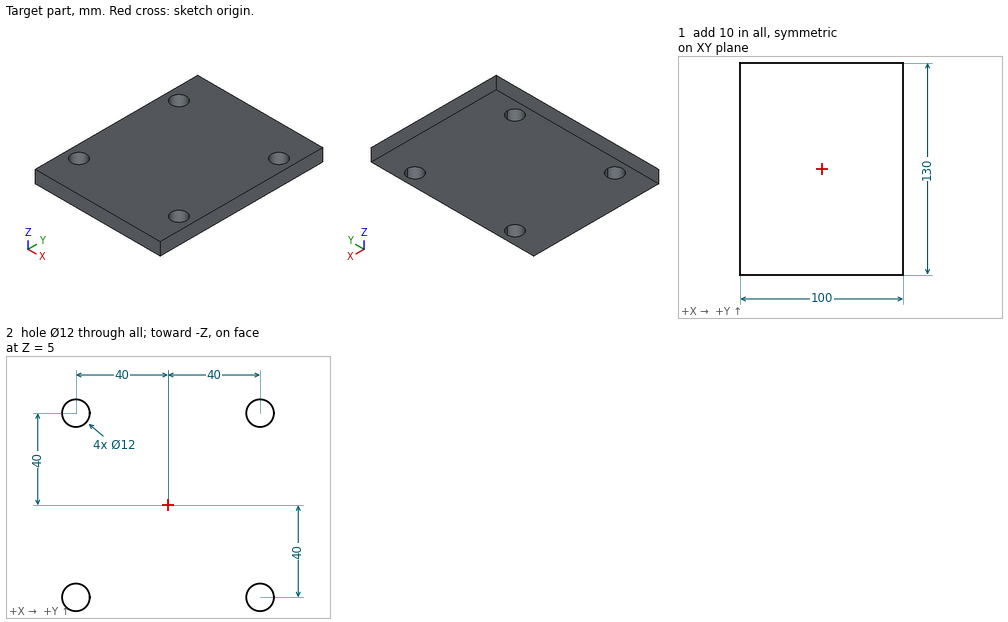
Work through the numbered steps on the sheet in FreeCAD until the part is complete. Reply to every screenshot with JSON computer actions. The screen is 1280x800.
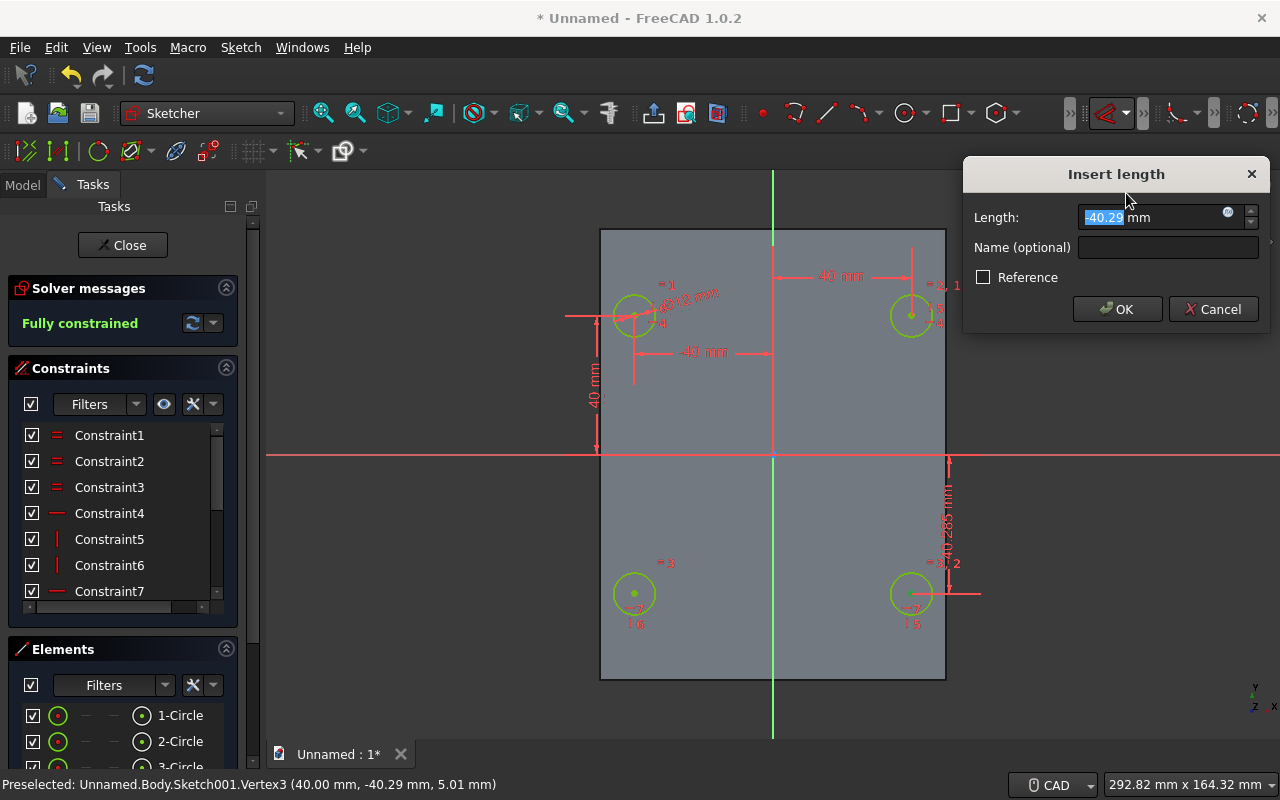
{"action": "type", "text": "-40"}
{"action": "key", "text": "Return"}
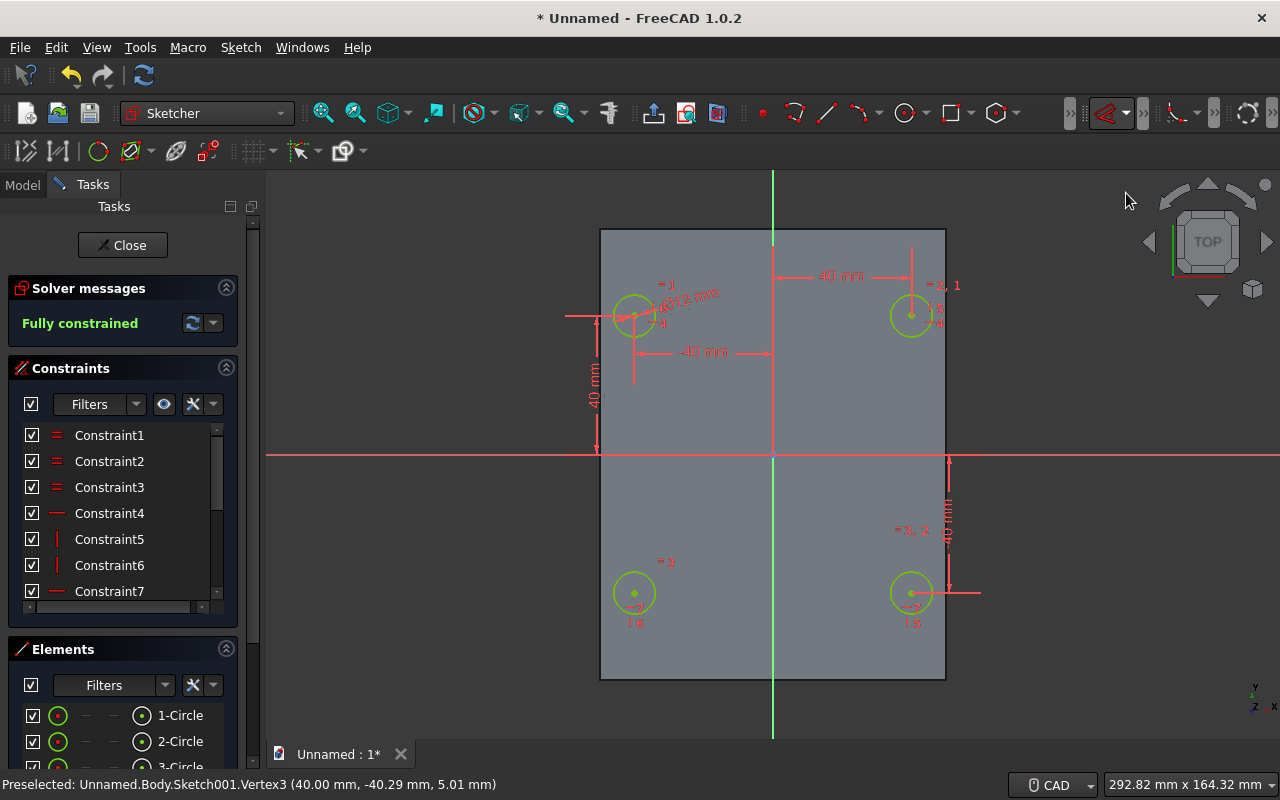
{"action": "left_click", "coordinate": [123, 245]}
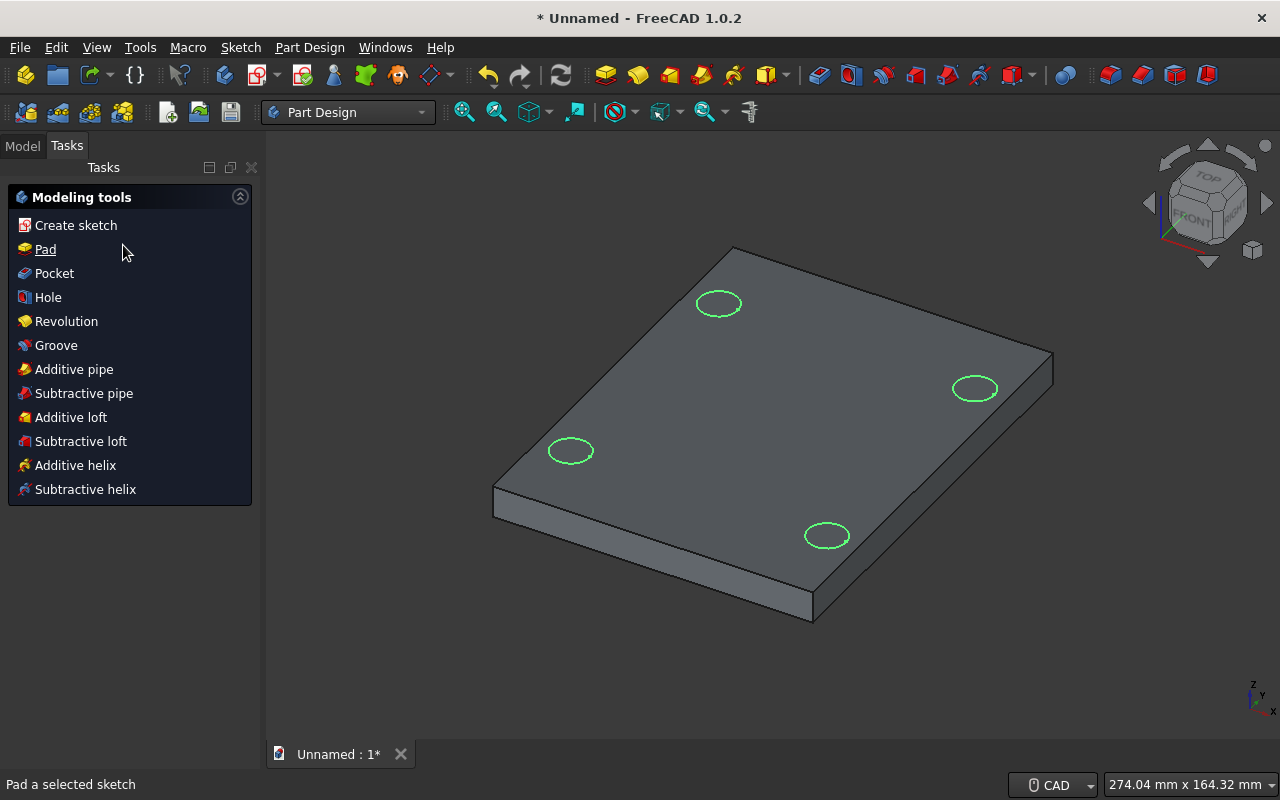
{"action": "left_click", "coordinate": [852, 76]}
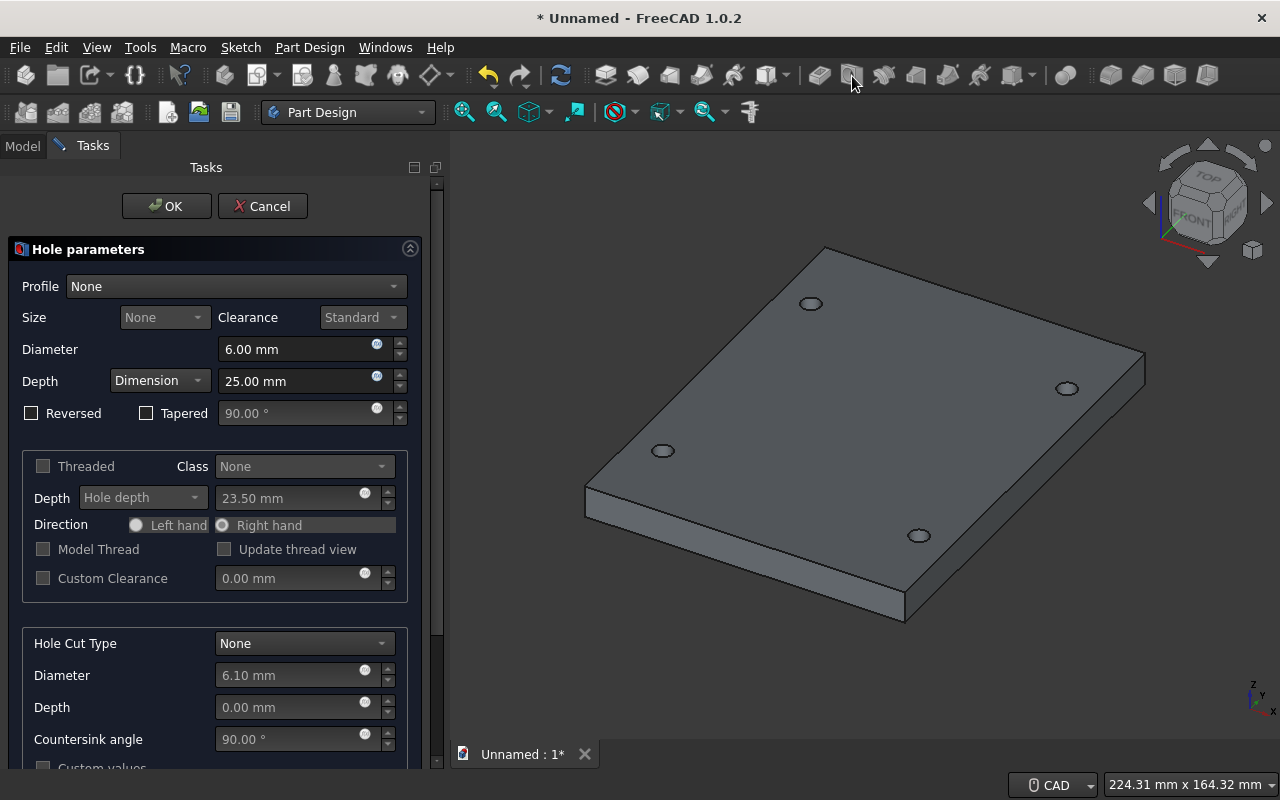
{"action": "triple_click", "coordinate": [305, 349]}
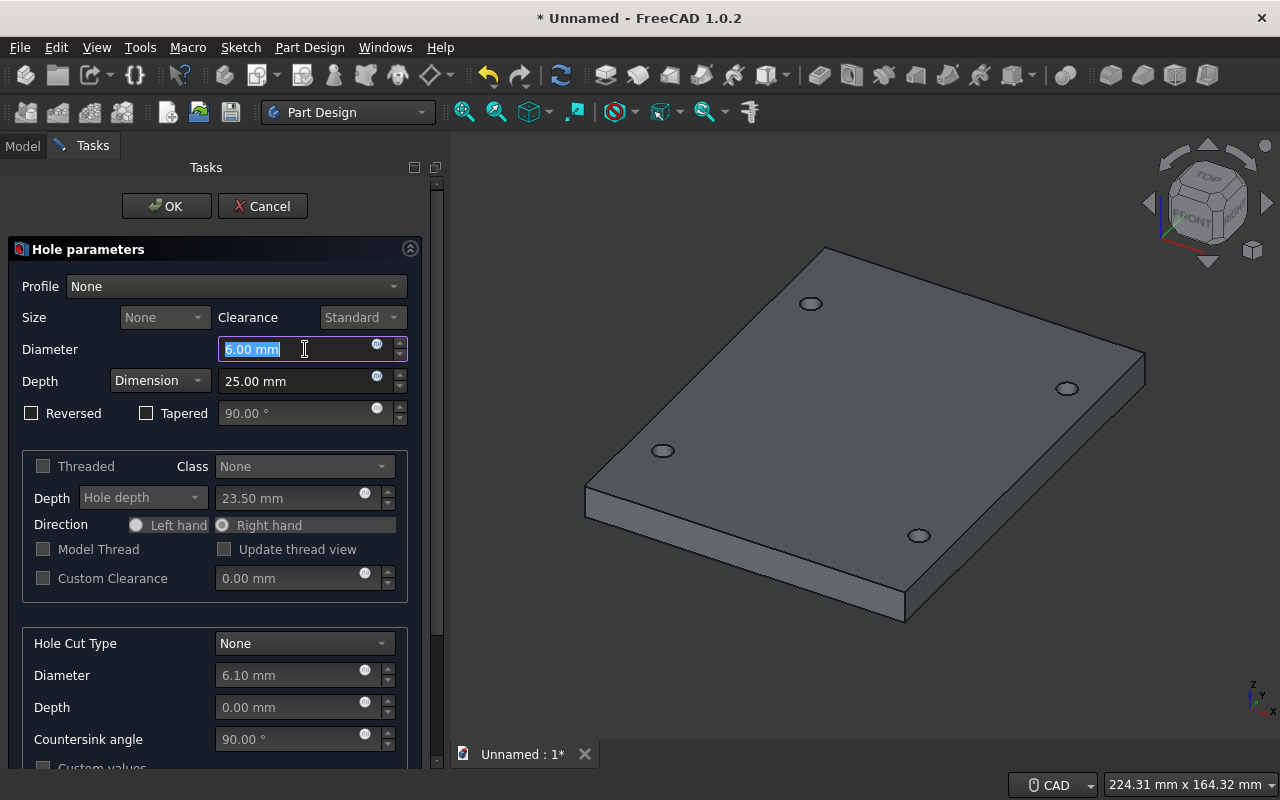
{"action": "type", "text": "12"}
{"action": "key", "text": "Tab"}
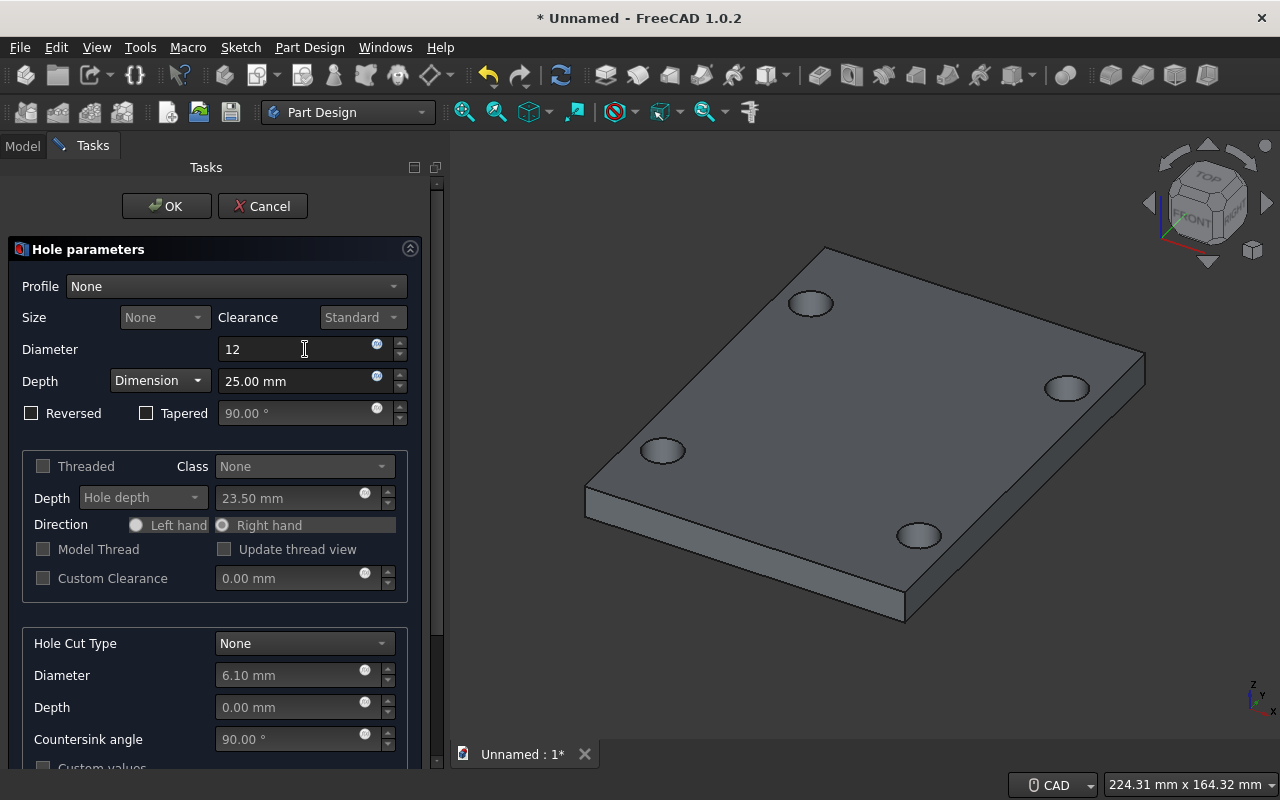
{"action": "left_click", "coordinate": [161, 380]}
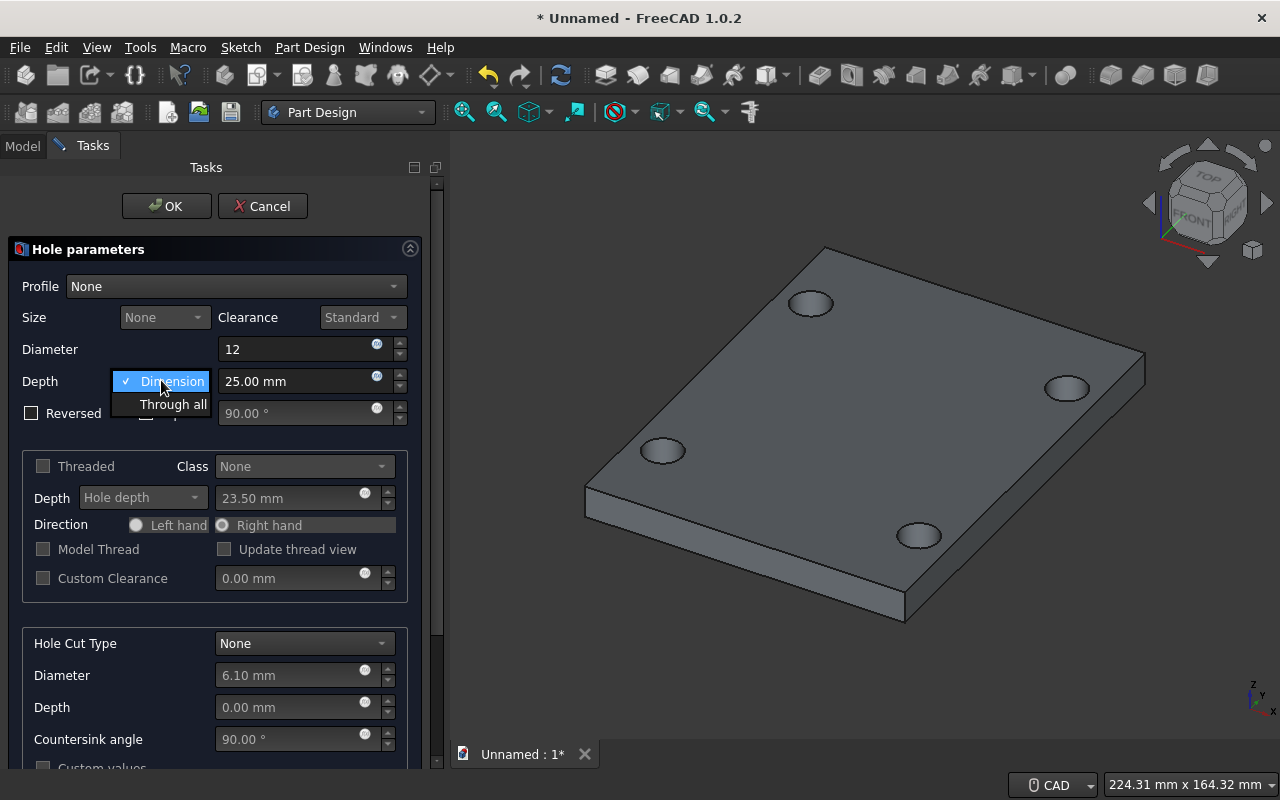
{"action": "left_click", "coordinate": [160, 404]}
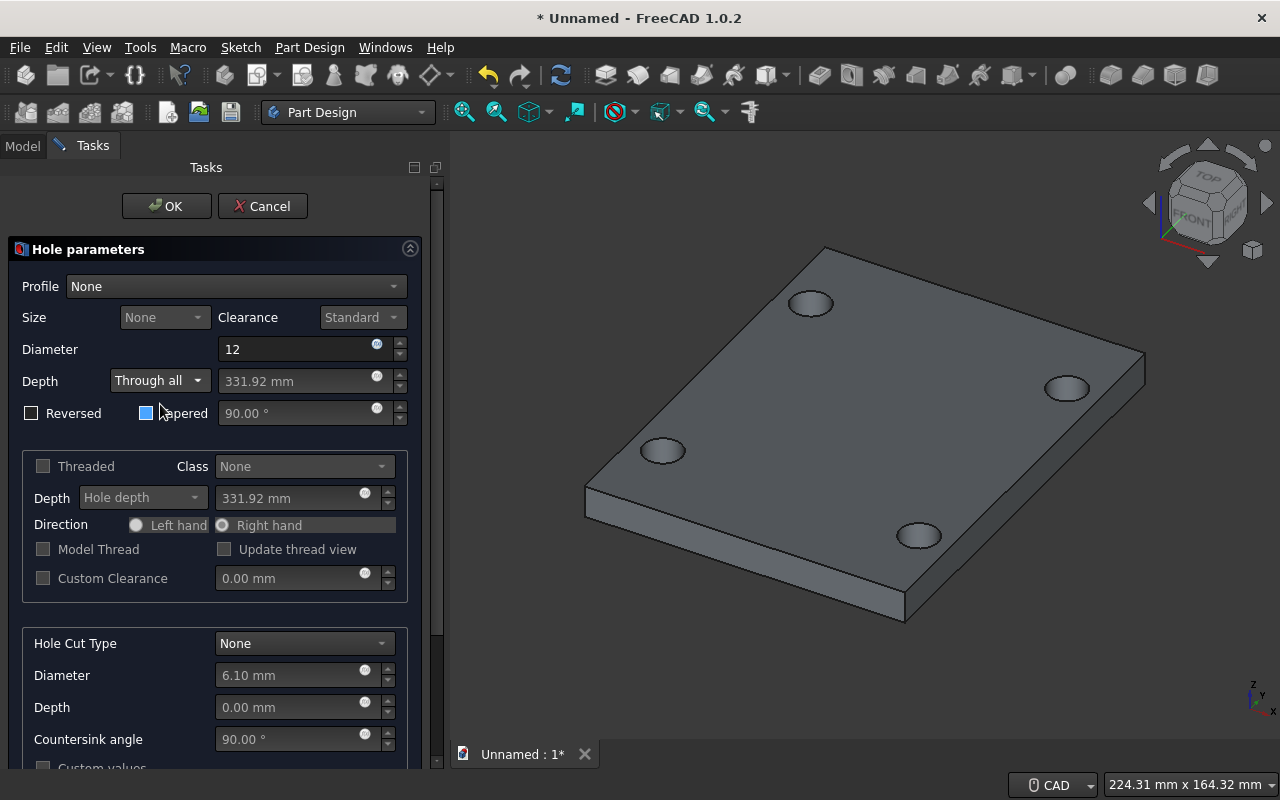
{"action": "left_click", "coordinate": [167, 206]}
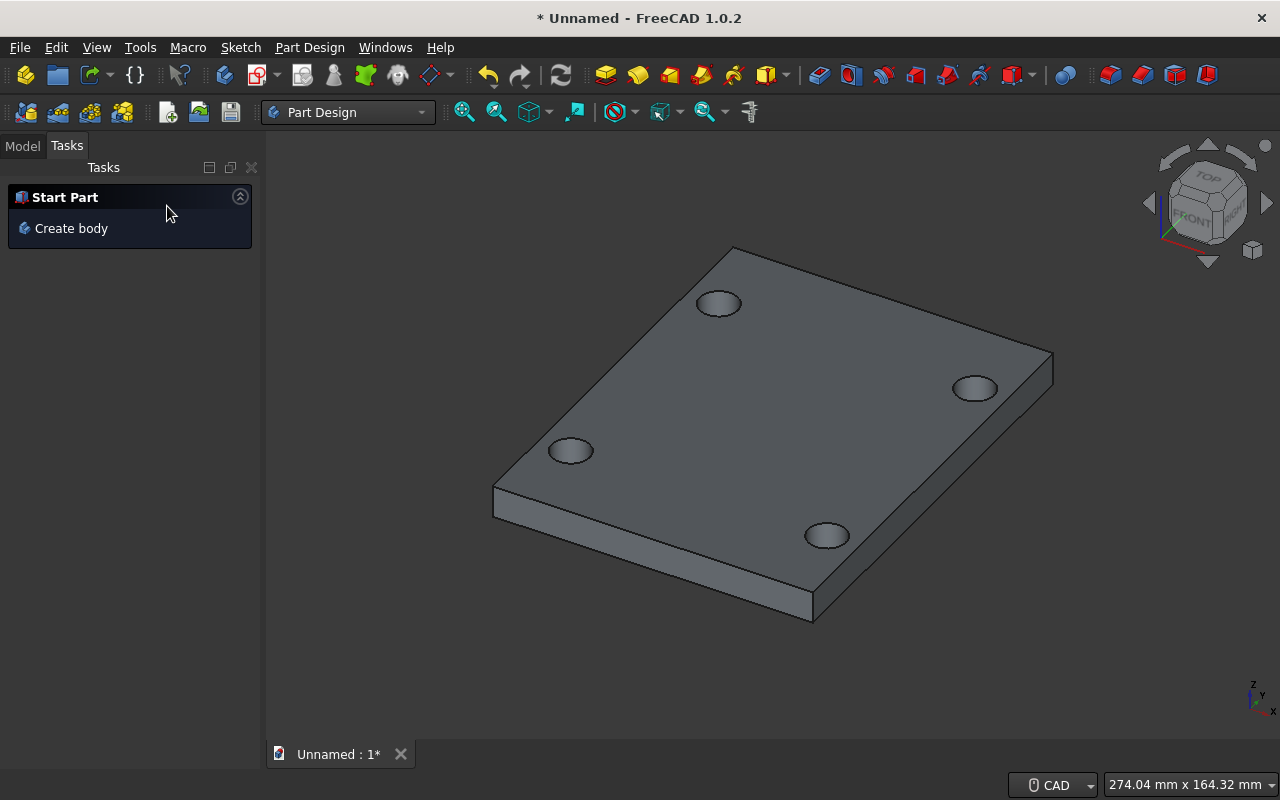
{"action": "key", "text": "0"}